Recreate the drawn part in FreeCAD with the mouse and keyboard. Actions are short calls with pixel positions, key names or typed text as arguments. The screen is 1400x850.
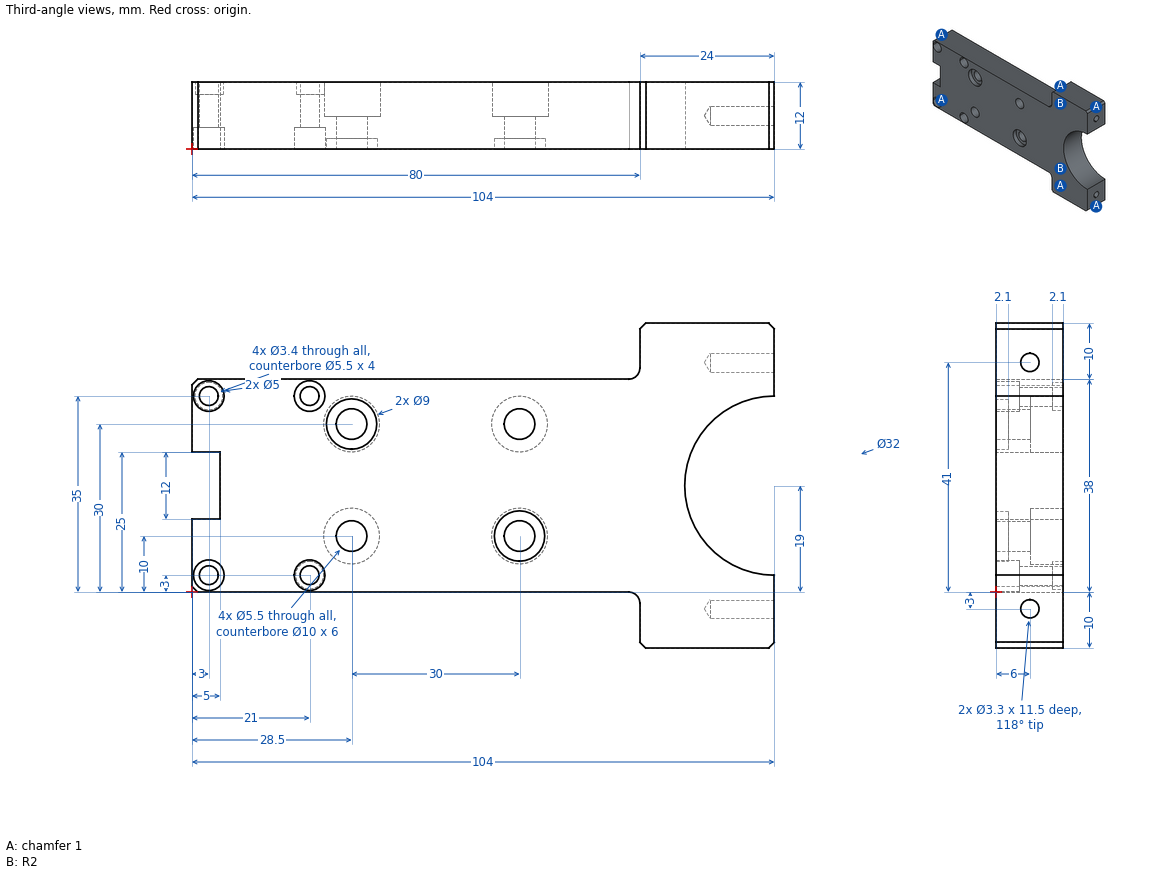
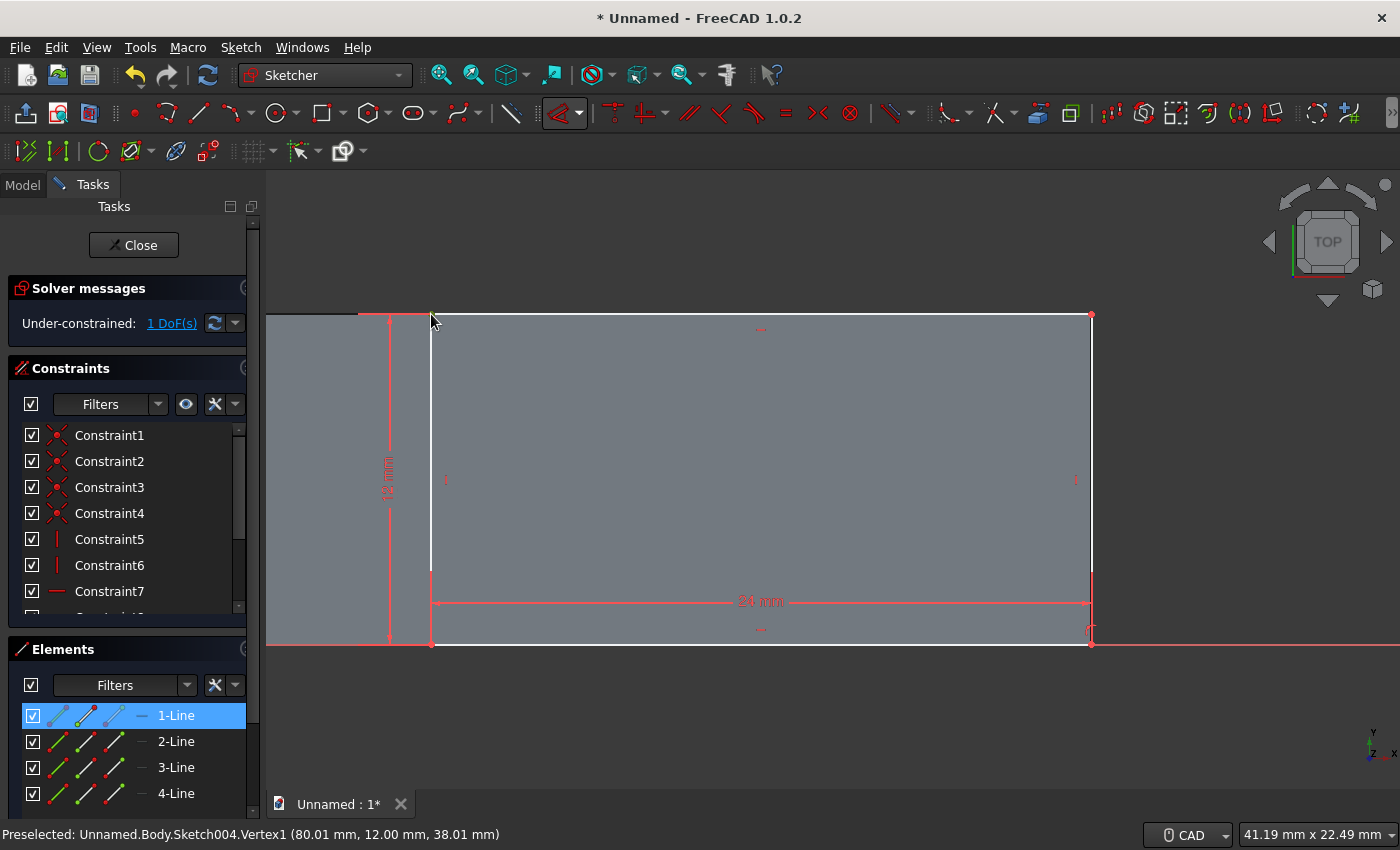
click(582, 114)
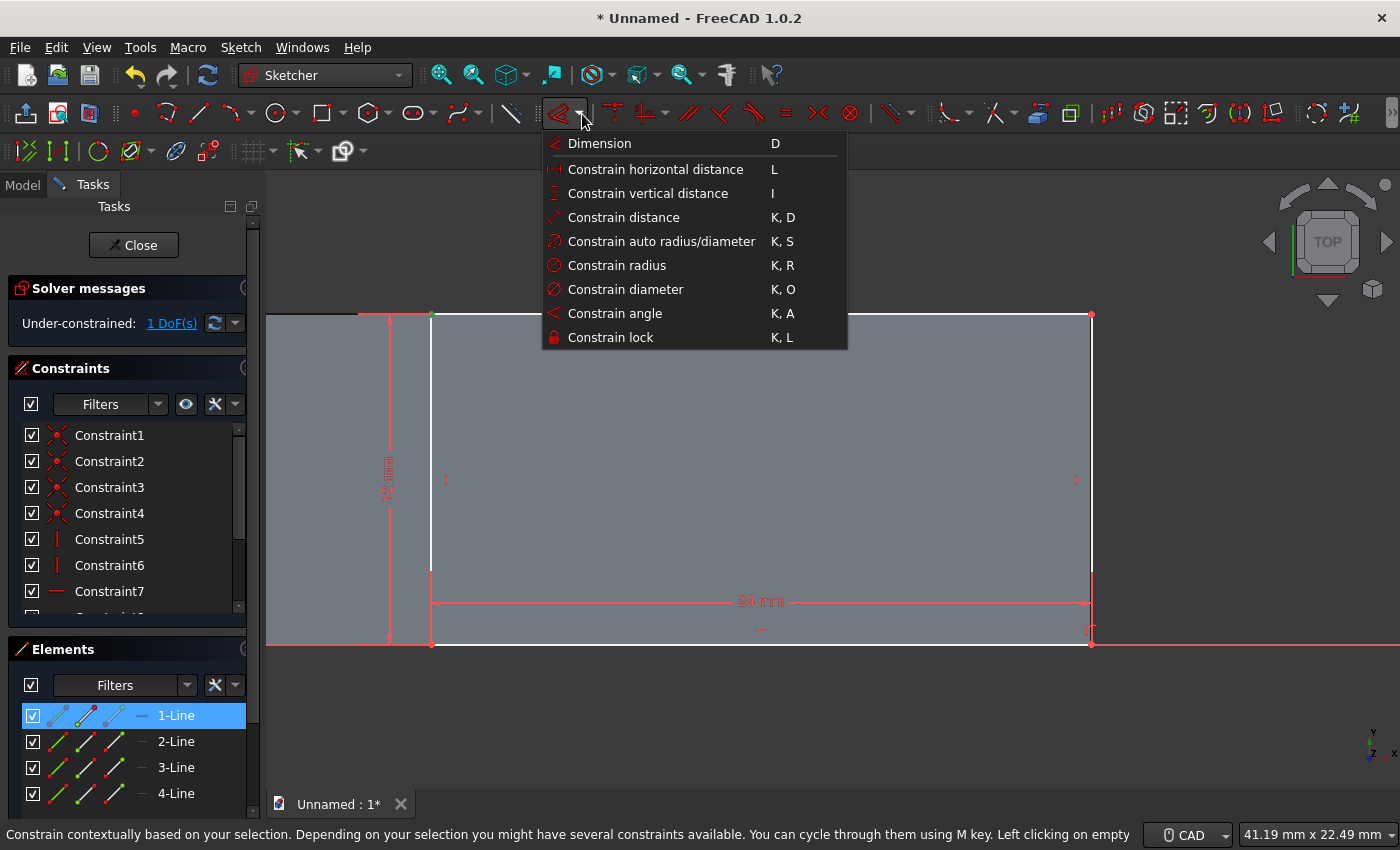
click(695, 169)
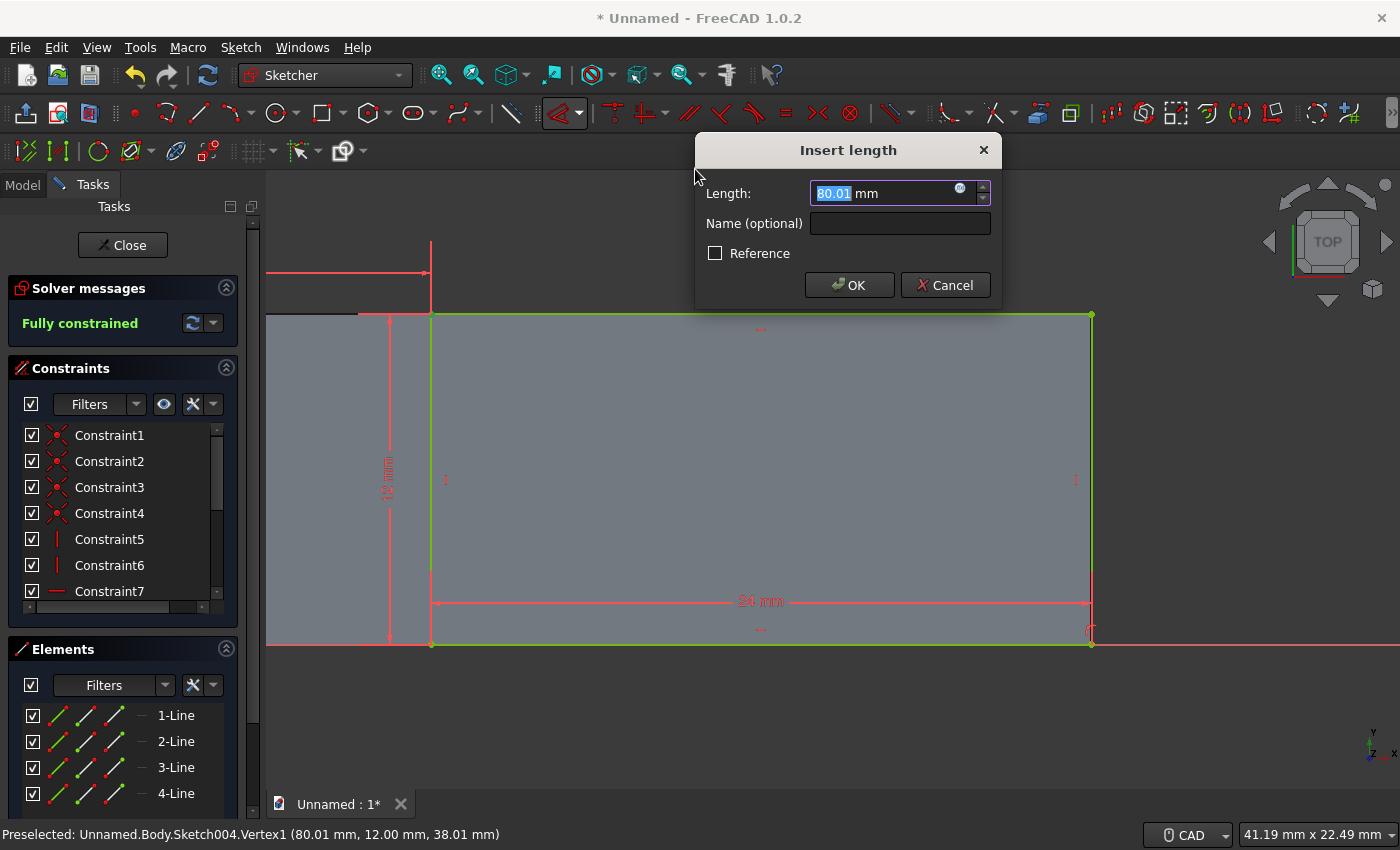
text(80)
key(Return)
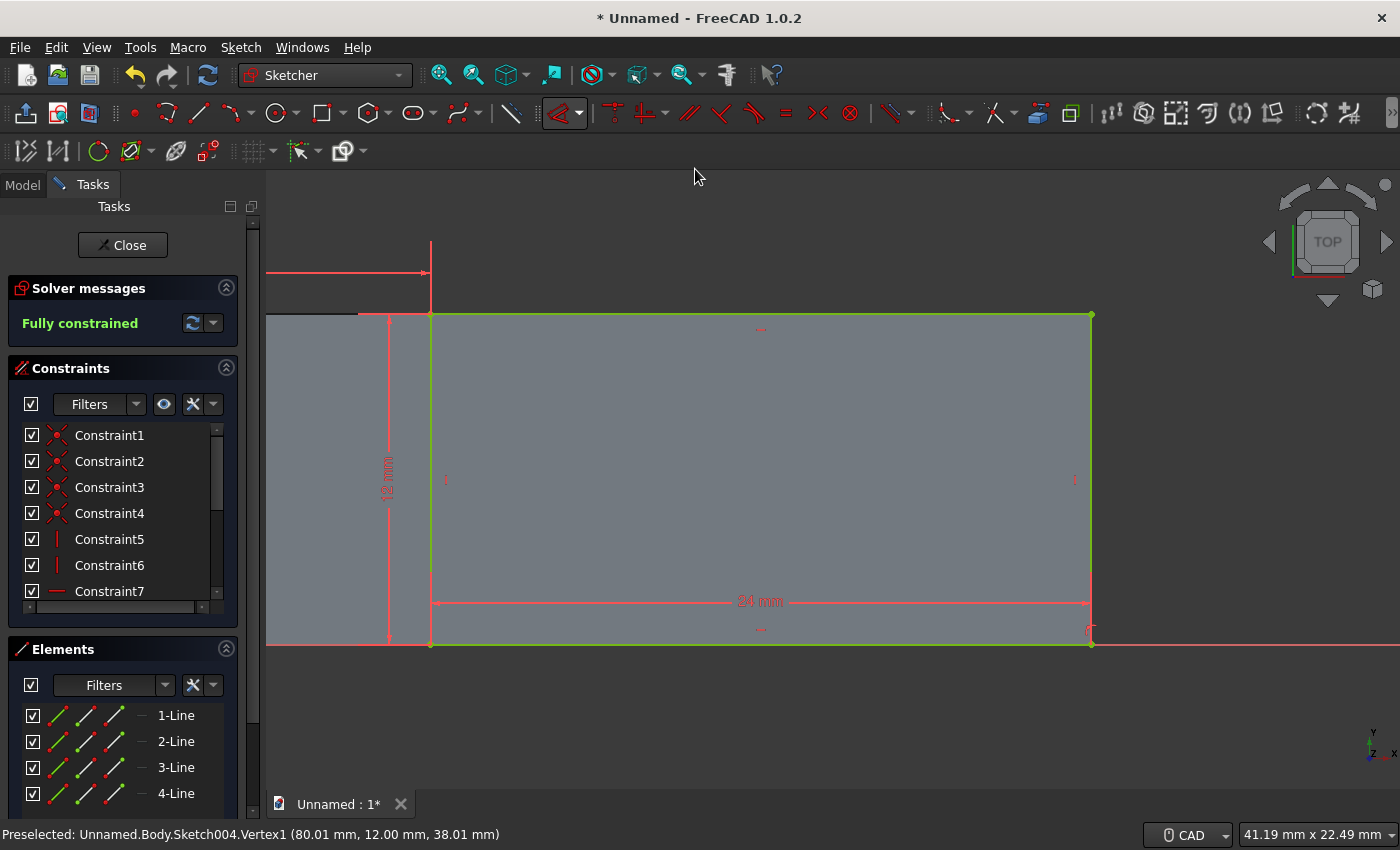
click(123, 245)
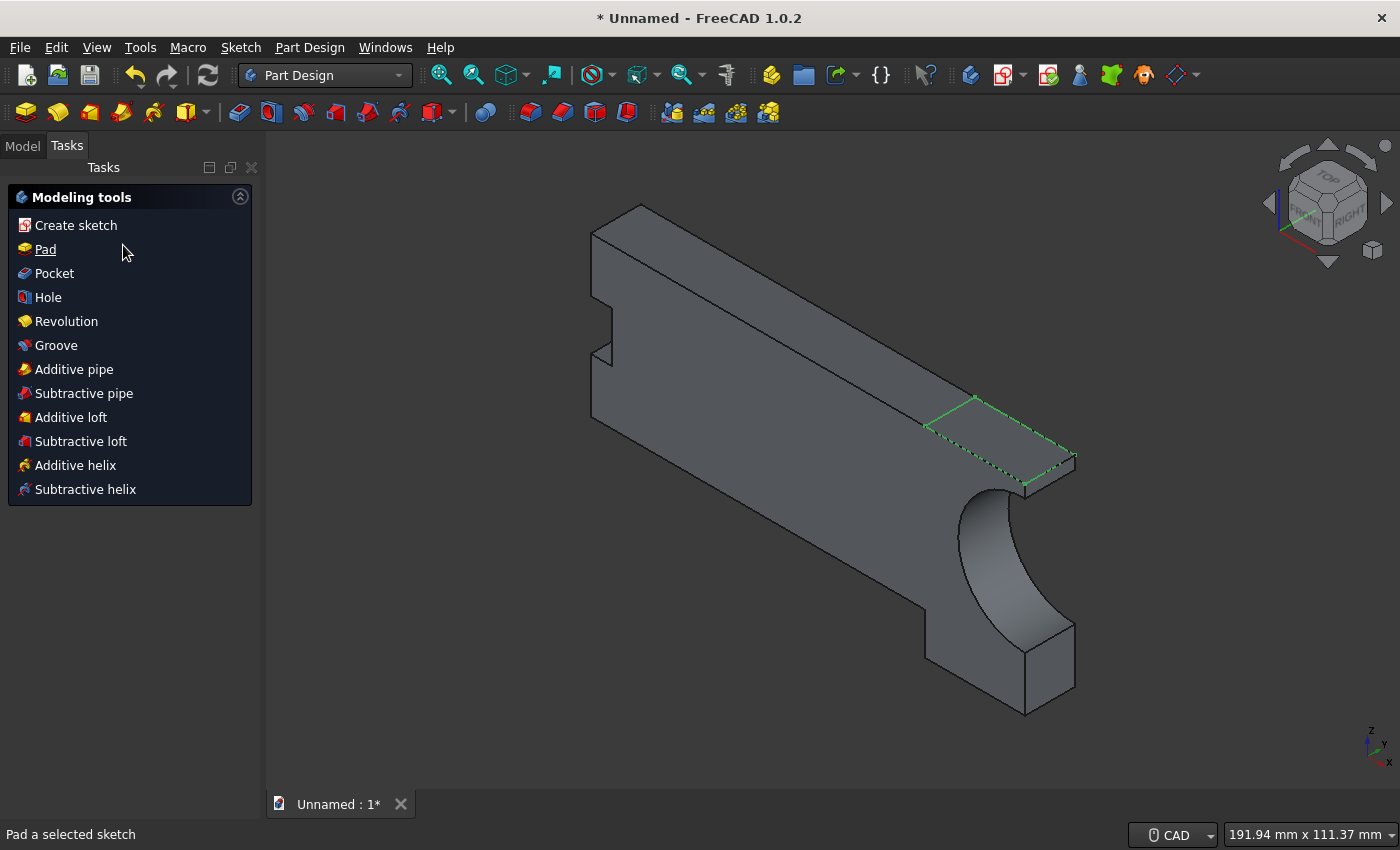
click(26, 112)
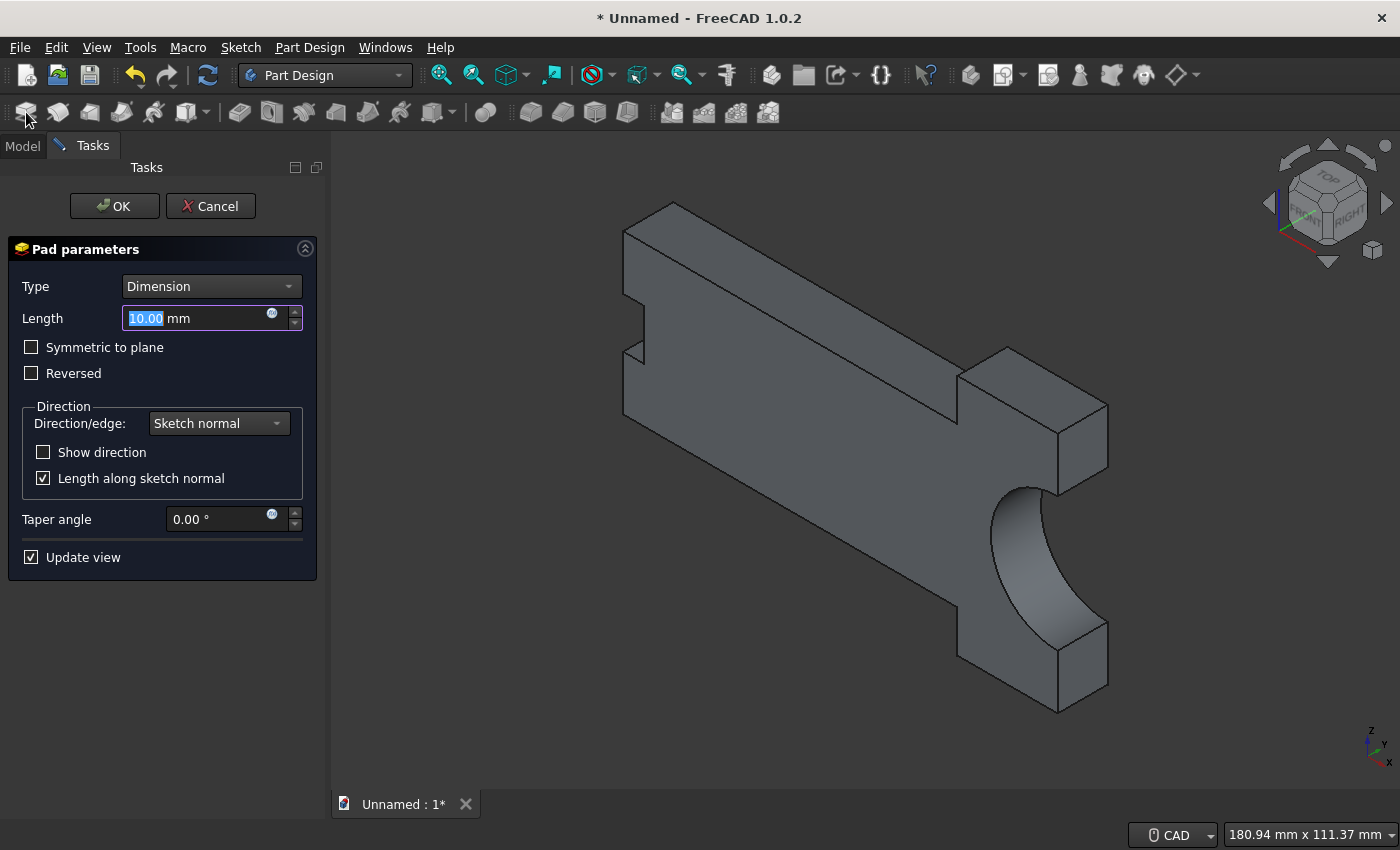
text(10)
key(Tab)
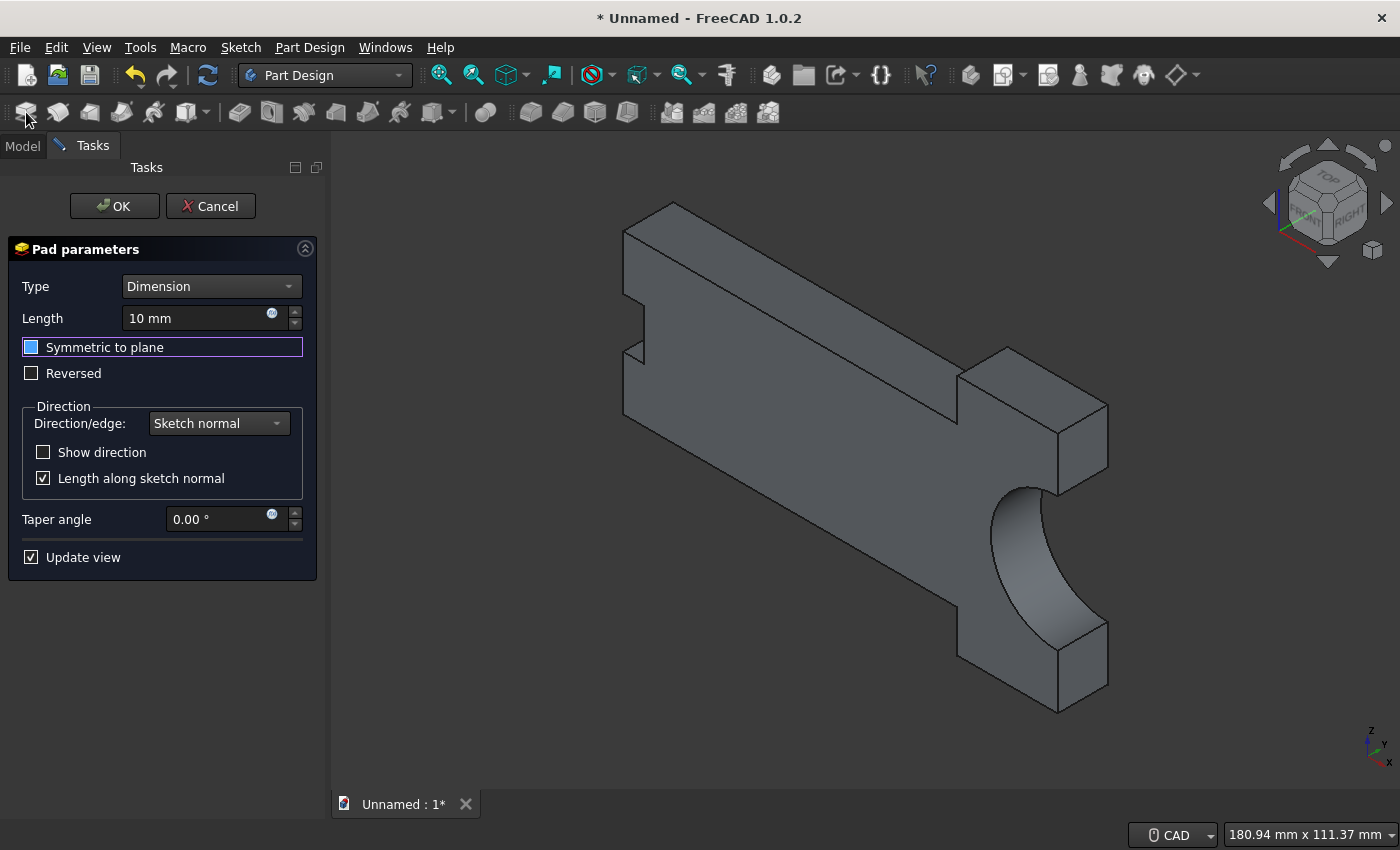
click(115, 206)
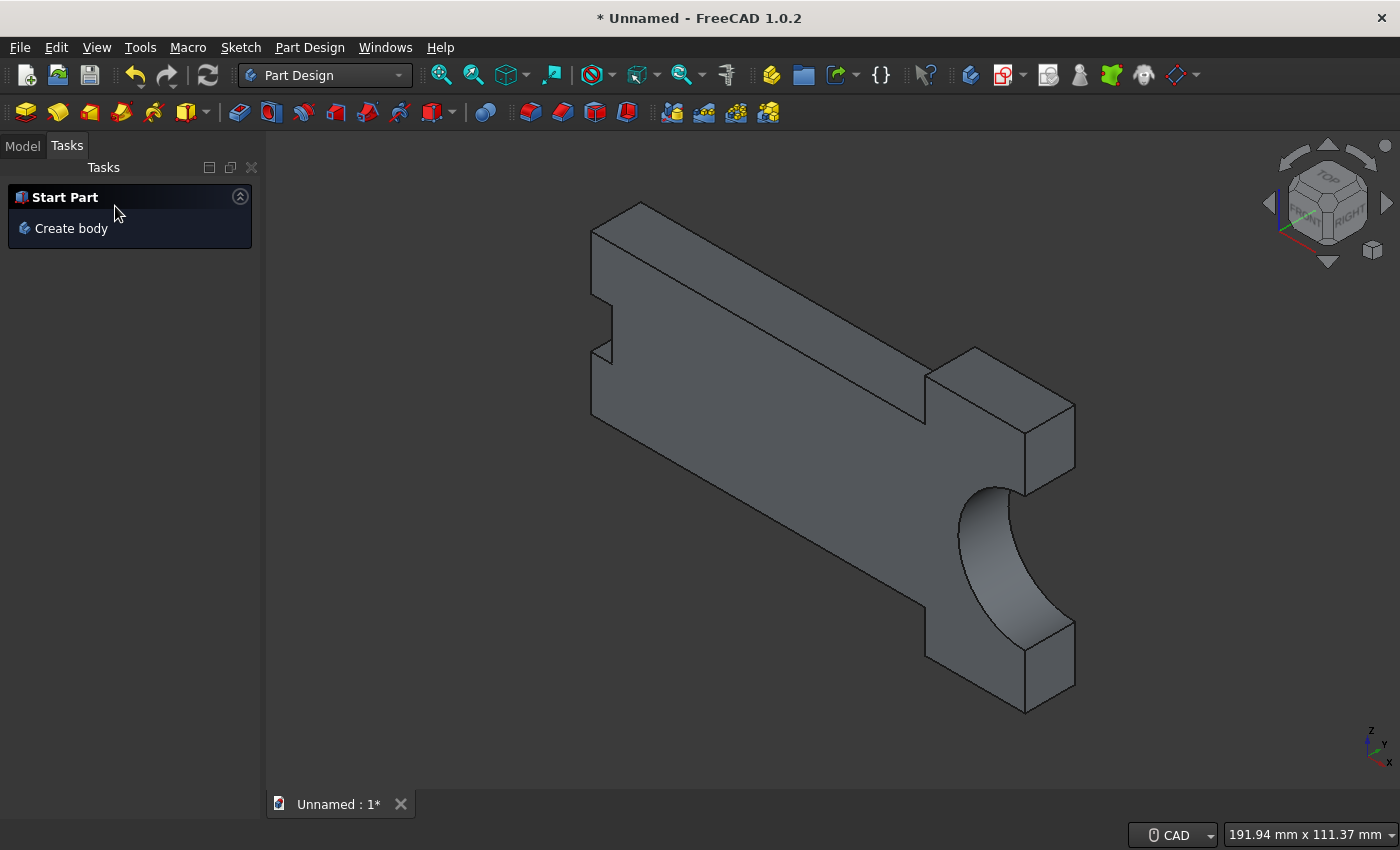
click(1050, 418)